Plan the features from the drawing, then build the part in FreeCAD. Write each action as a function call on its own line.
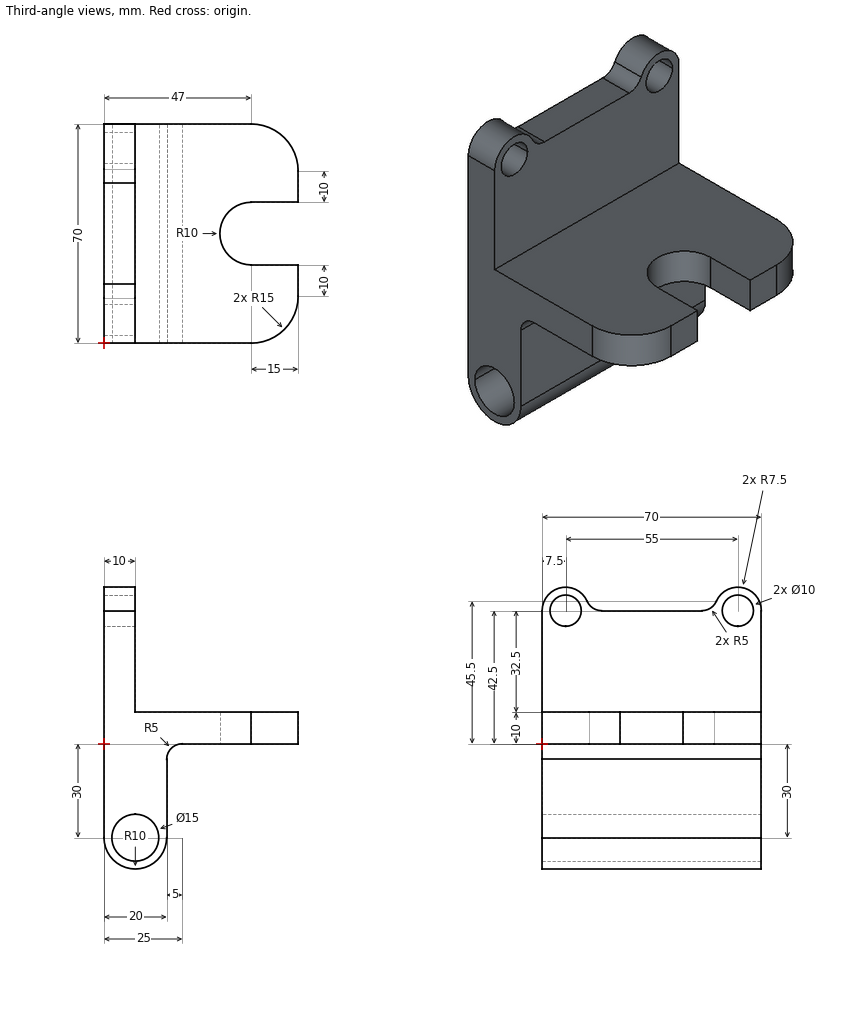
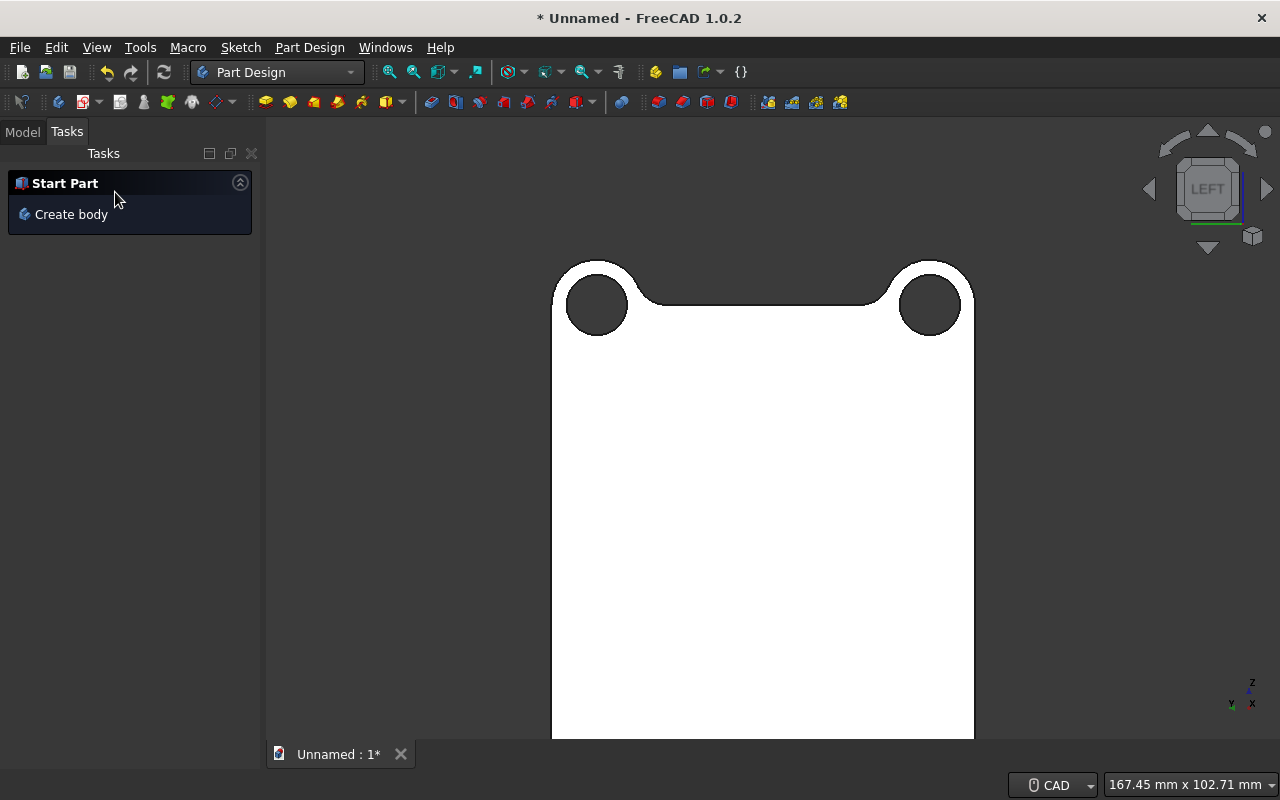
click(390, 72)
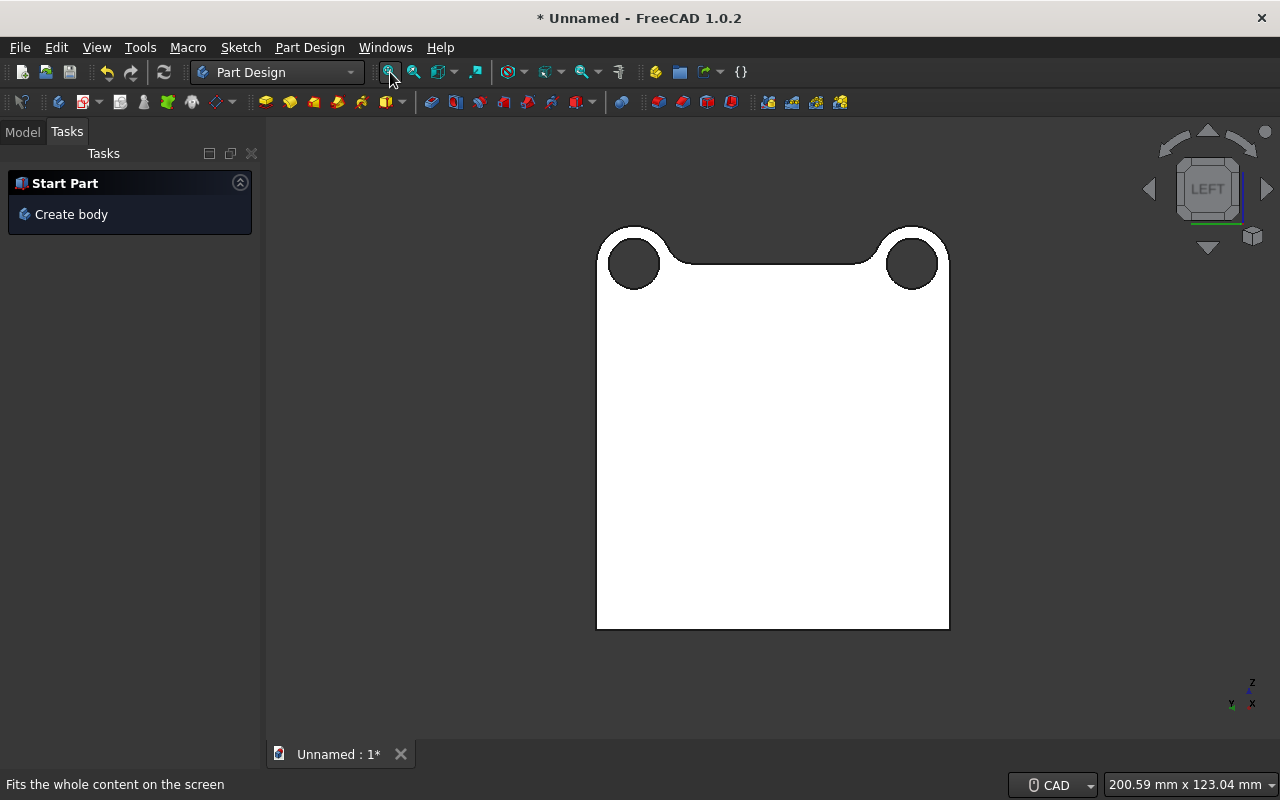
key(4)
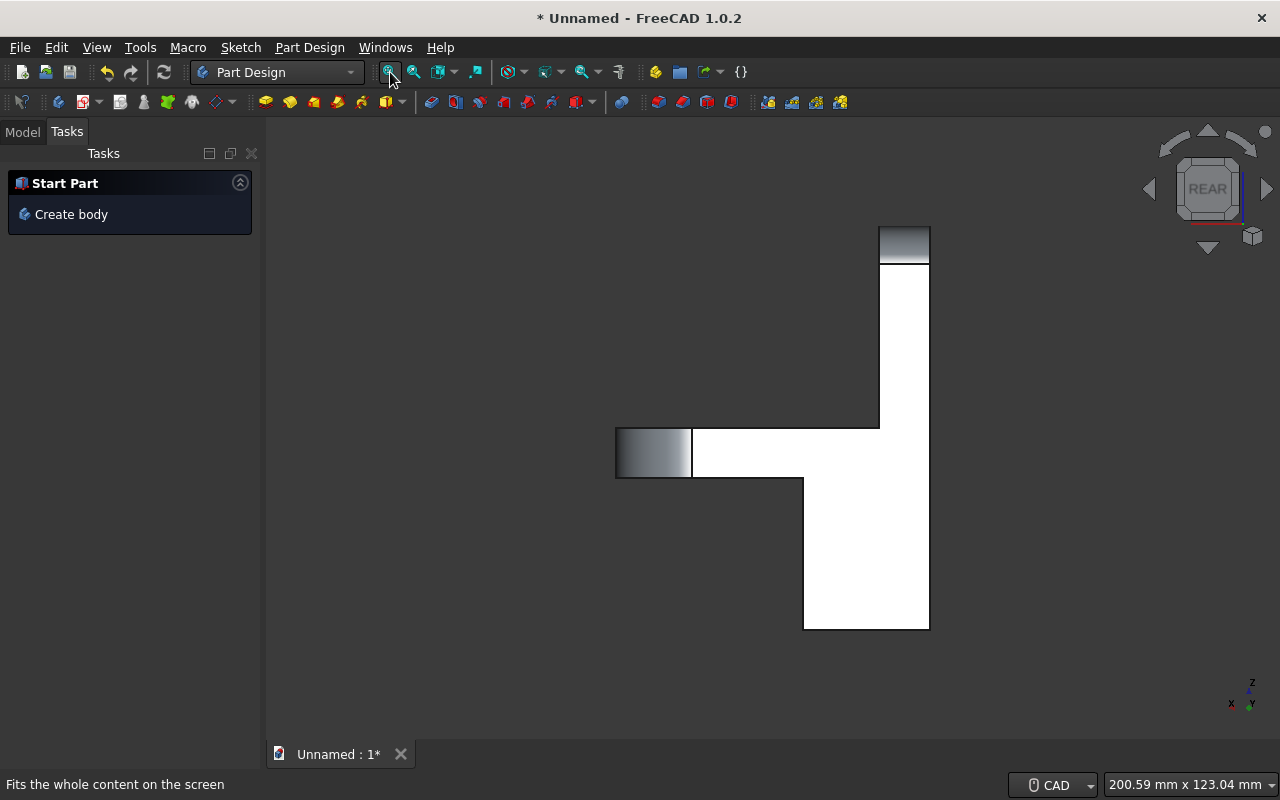
click(879, 498)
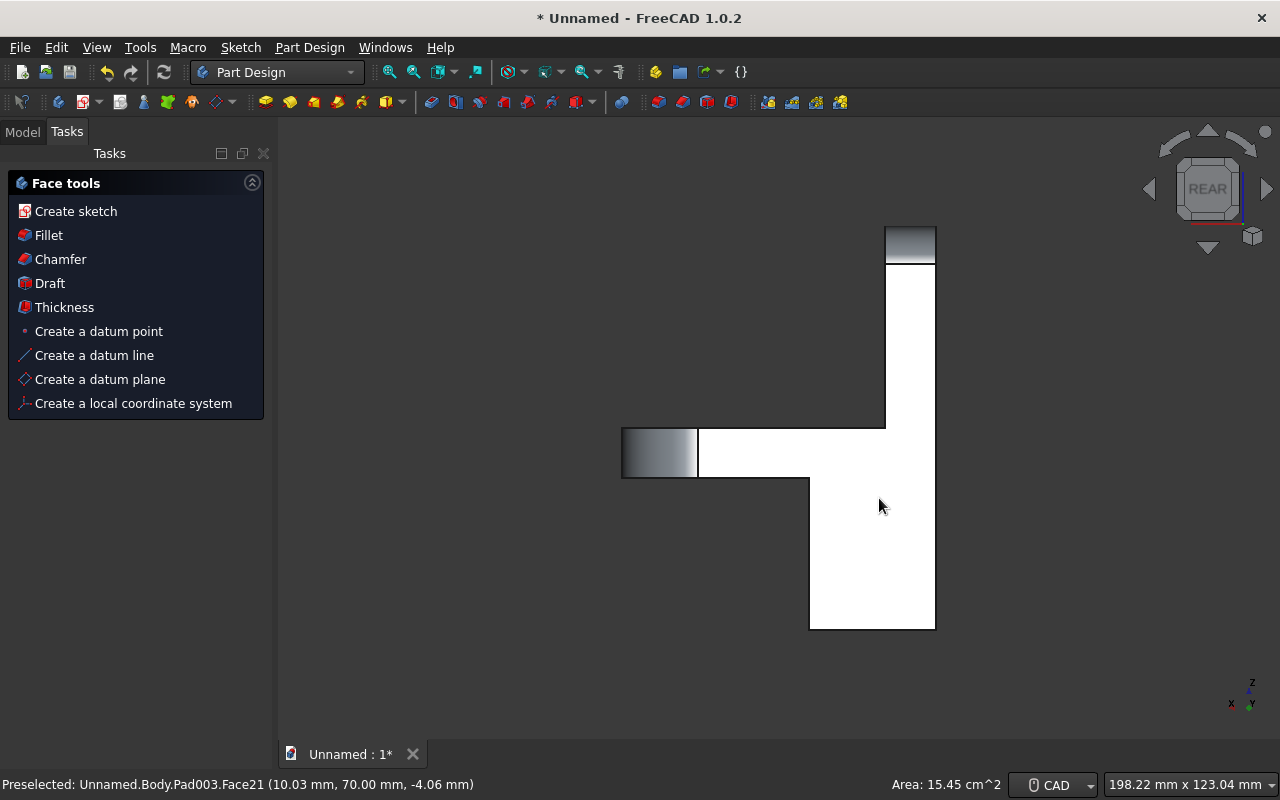
click(84, 102)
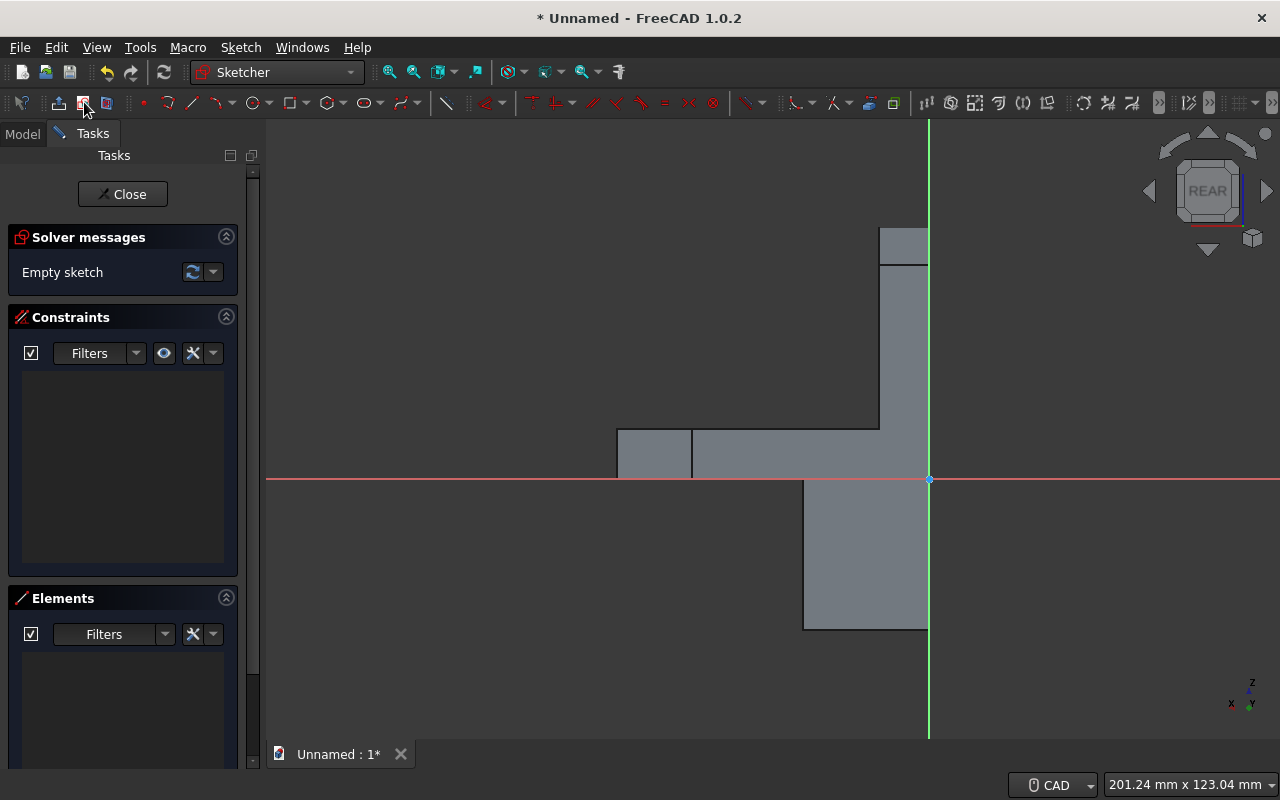
scroll(960, 628, up, 5)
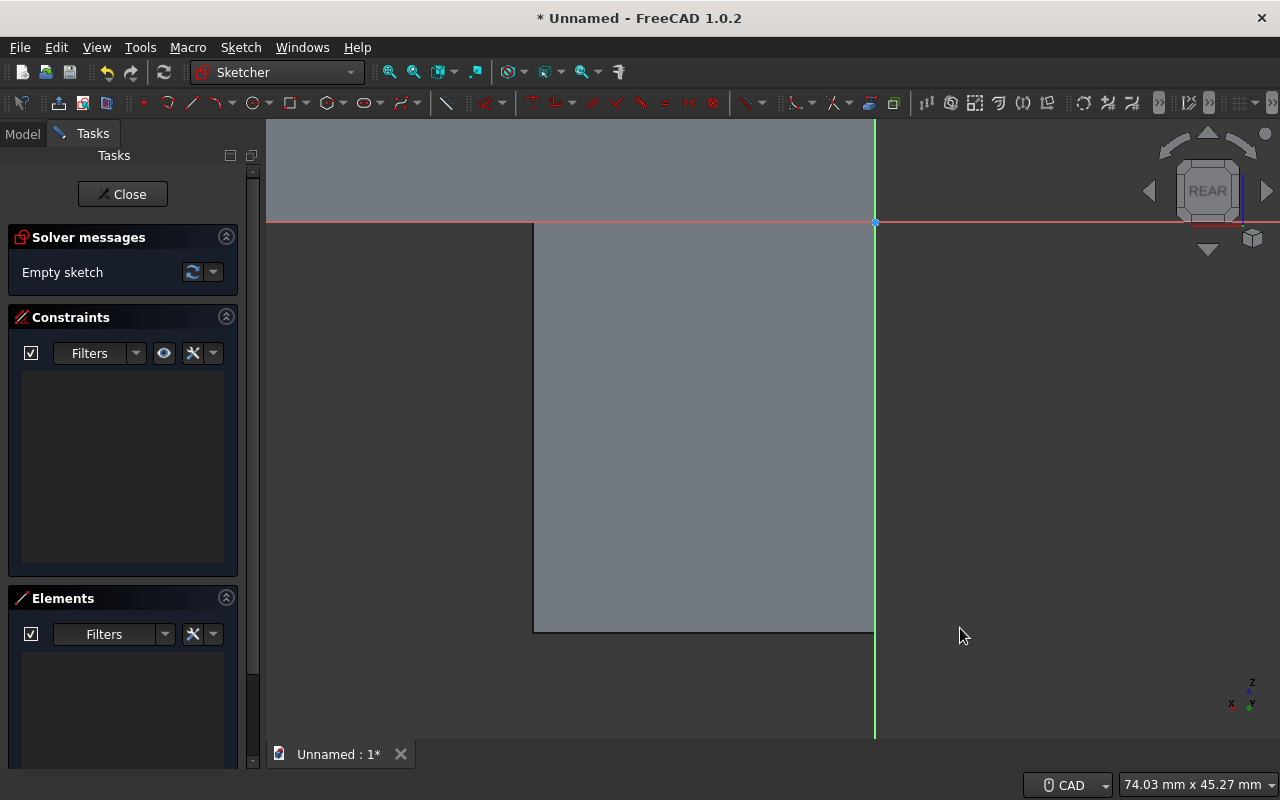
click(290, 104)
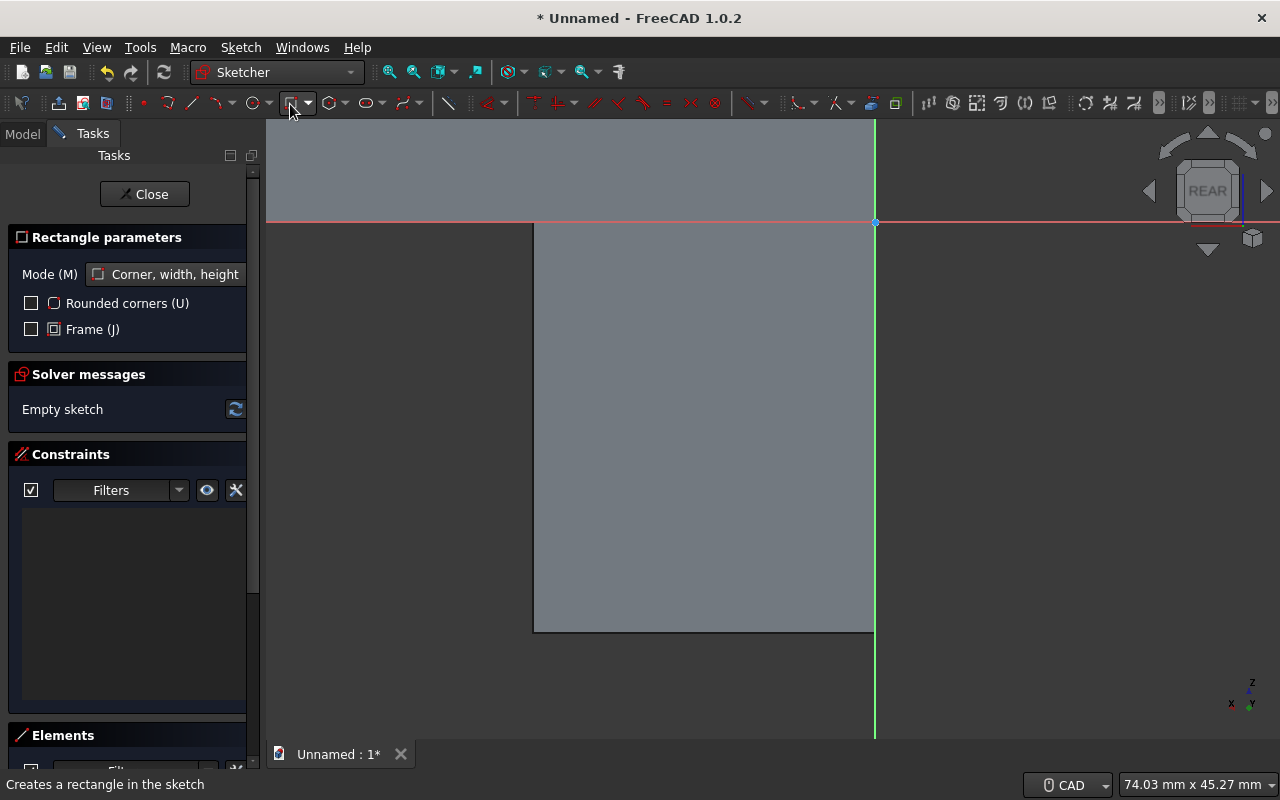
click(533, 222)
click(601, 633)
key(Escape)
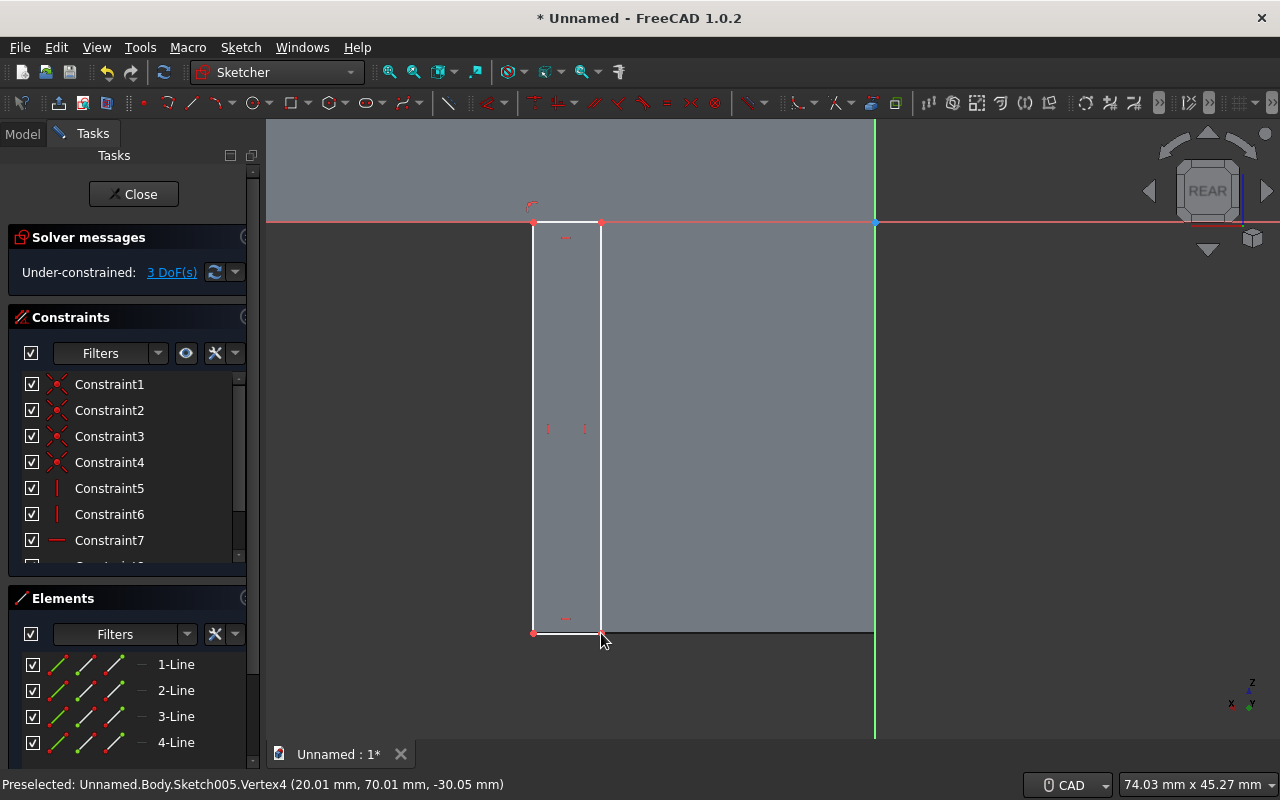
click(488, 104)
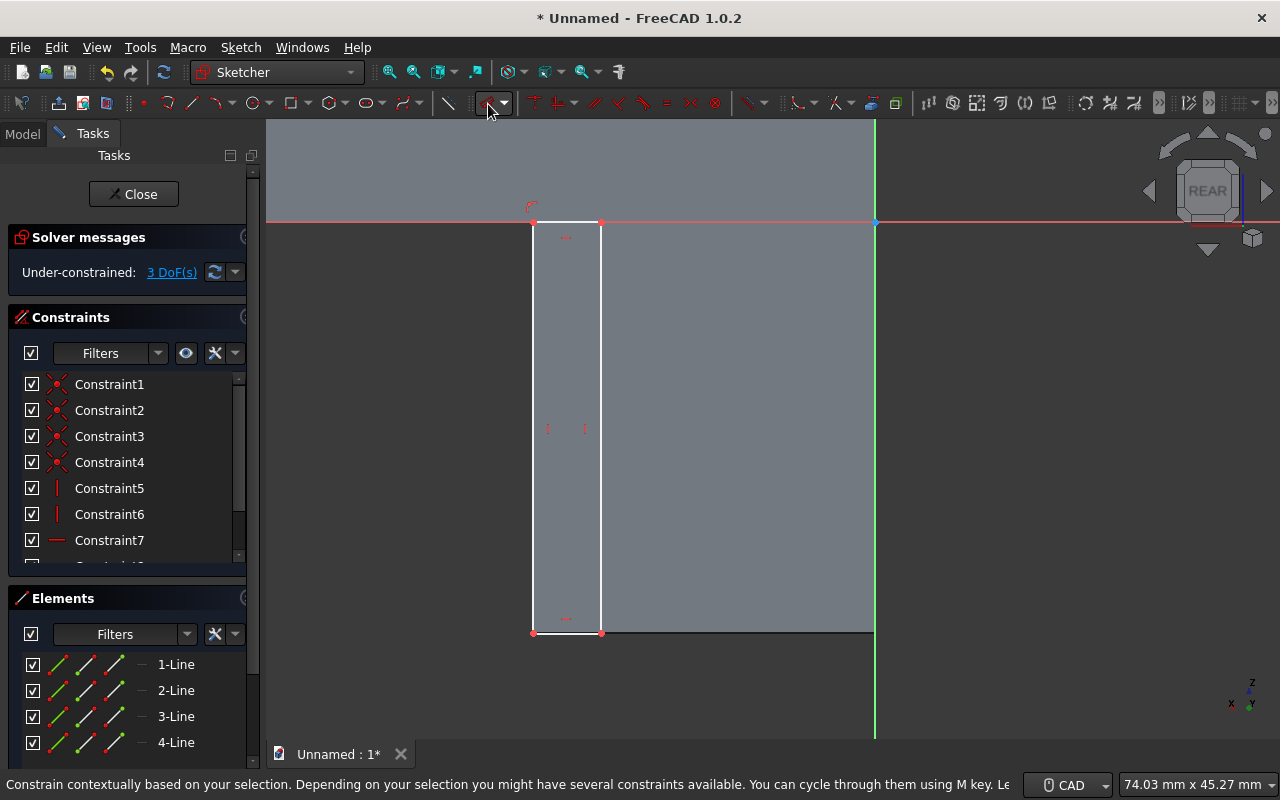
click(553, 634)
click(567, 668)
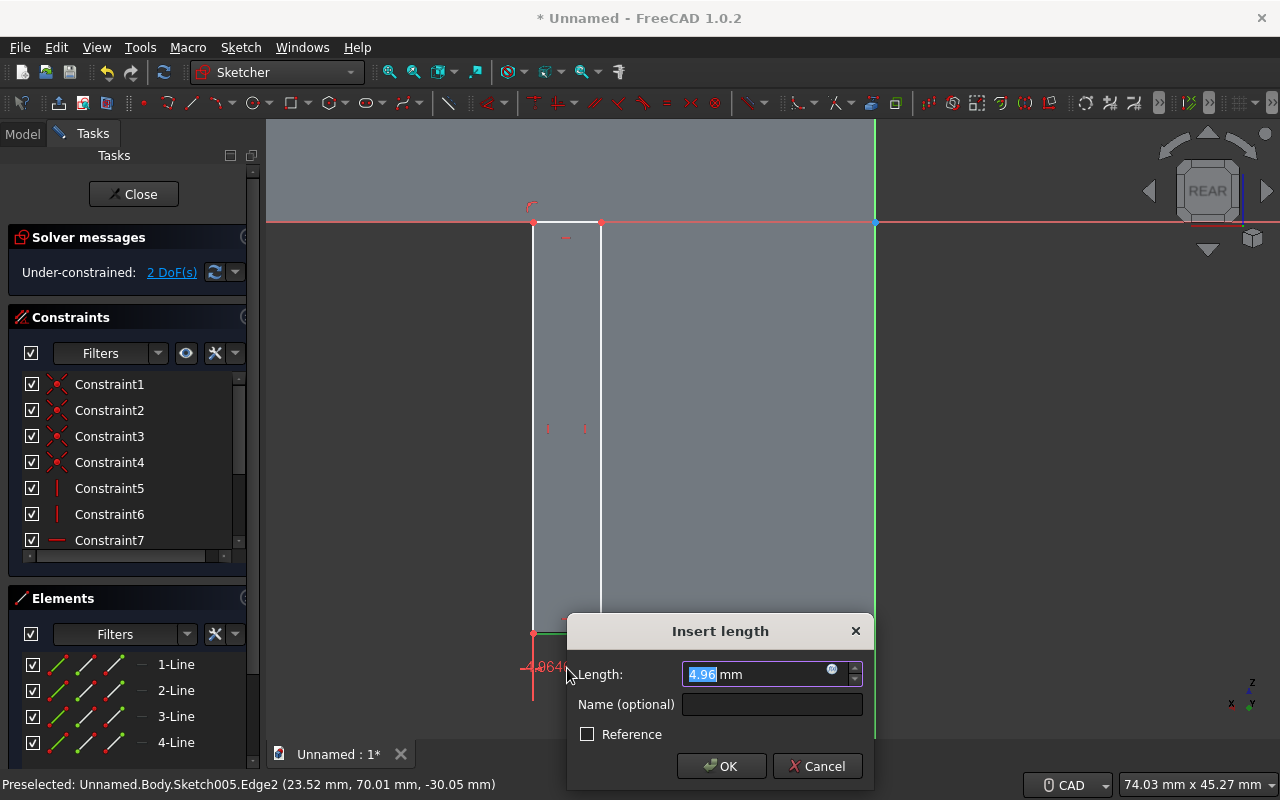
text(5)
key(Return)